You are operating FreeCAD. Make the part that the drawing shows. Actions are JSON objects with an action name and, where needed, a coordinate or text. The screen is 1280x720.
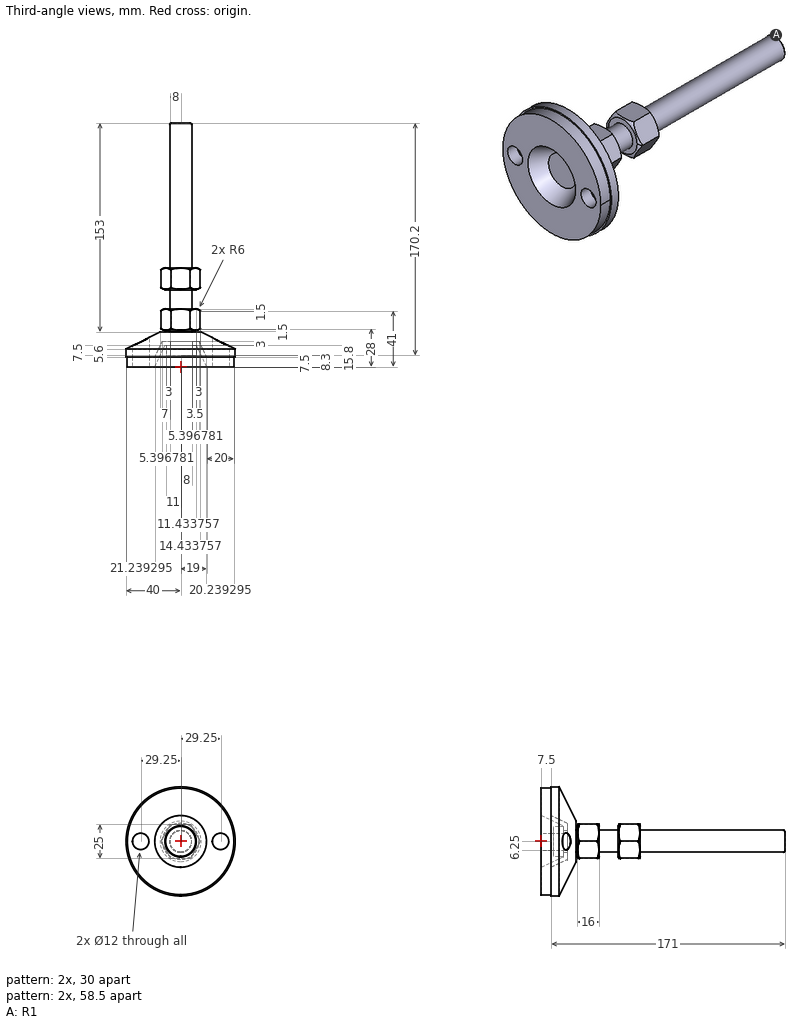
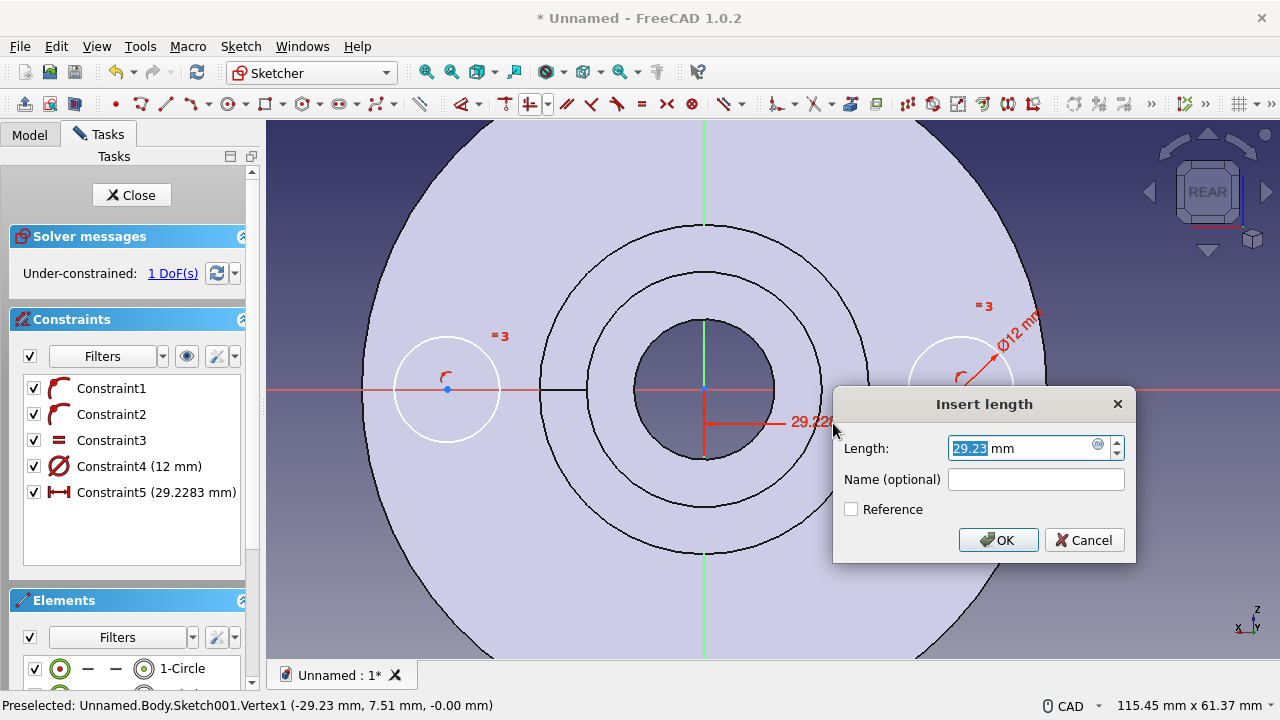
{"action": "type", "text": "29.25"}
{"action": "key", "text": "Return"}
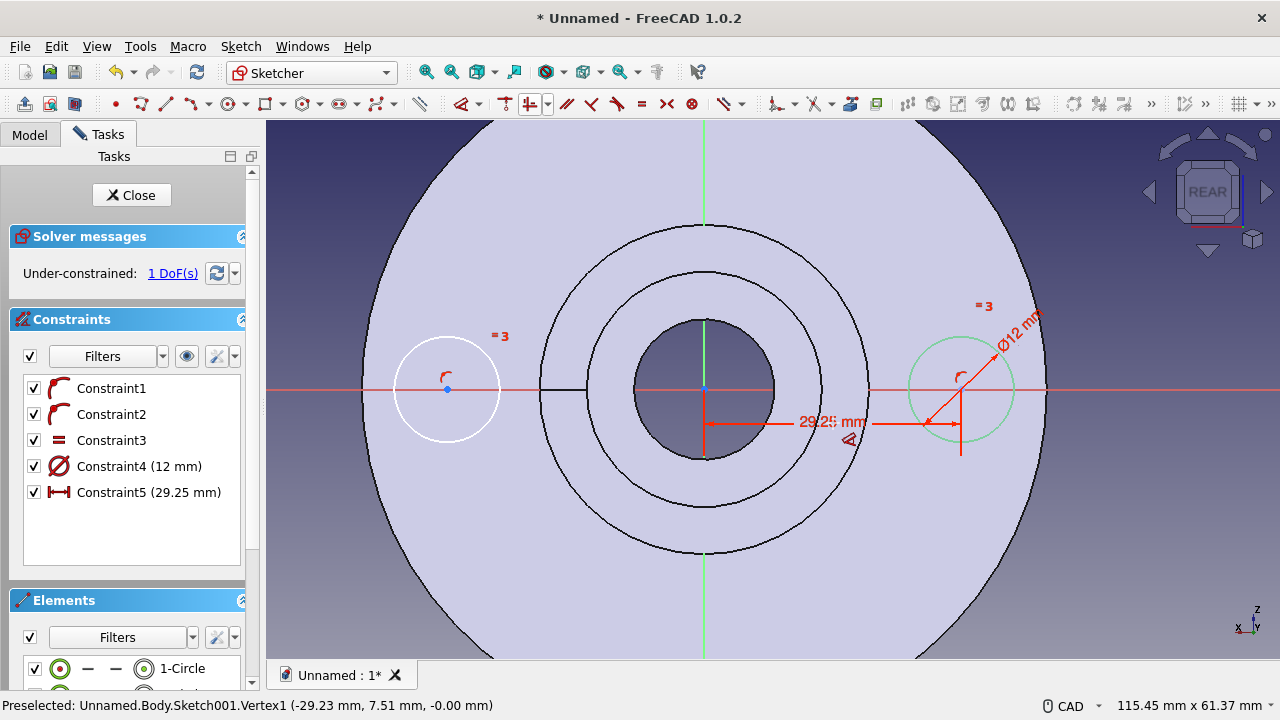
{"action": "left_click", "coordinate": [447, 389]}
{"action": "left_click", "coordinate": [576, 423]}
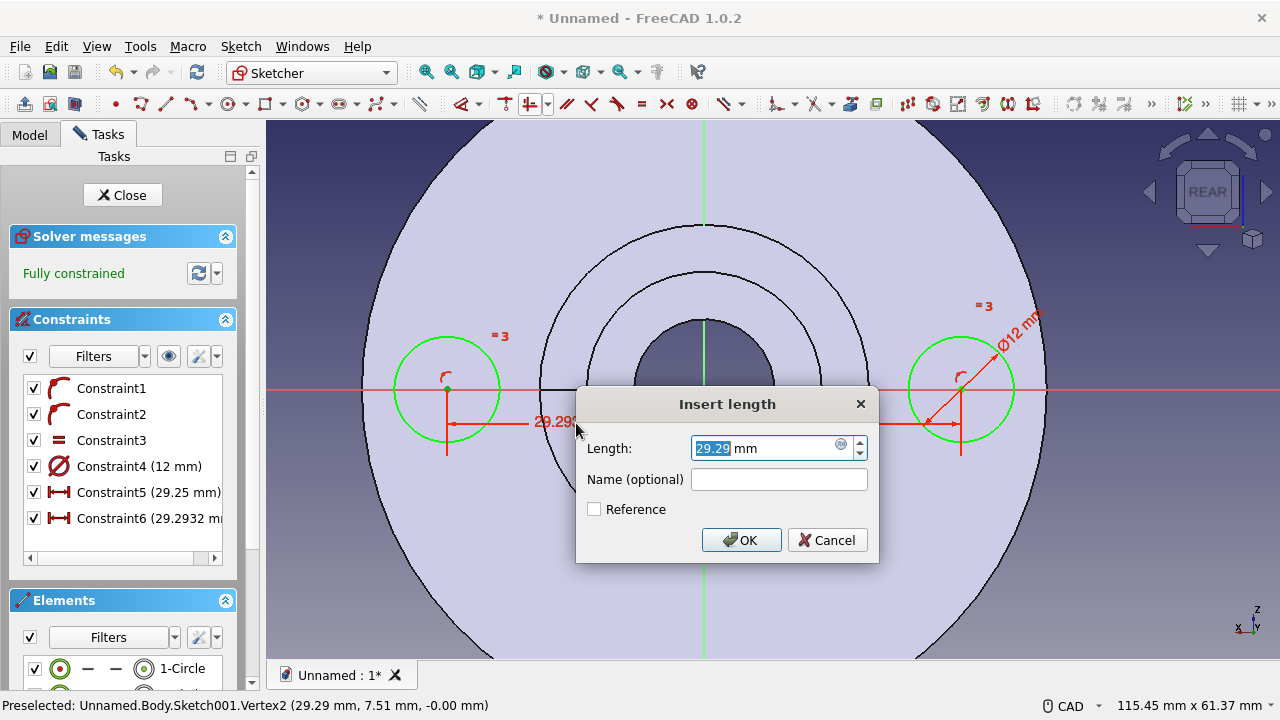
{"action": "type", "text": "29.25"}
{"action": "key", "text": "Return"}
{"action": "key", "text": "Escape"}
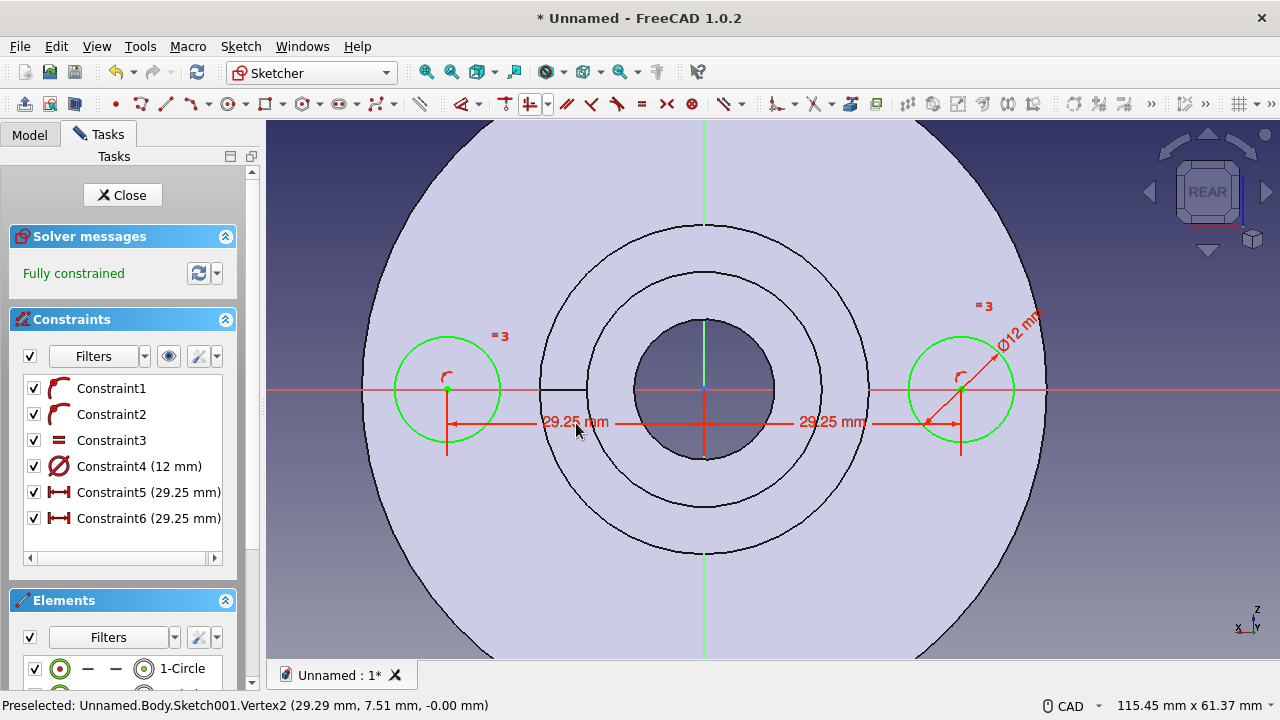
{"action": "left_click", "coordinate": [123, 195]}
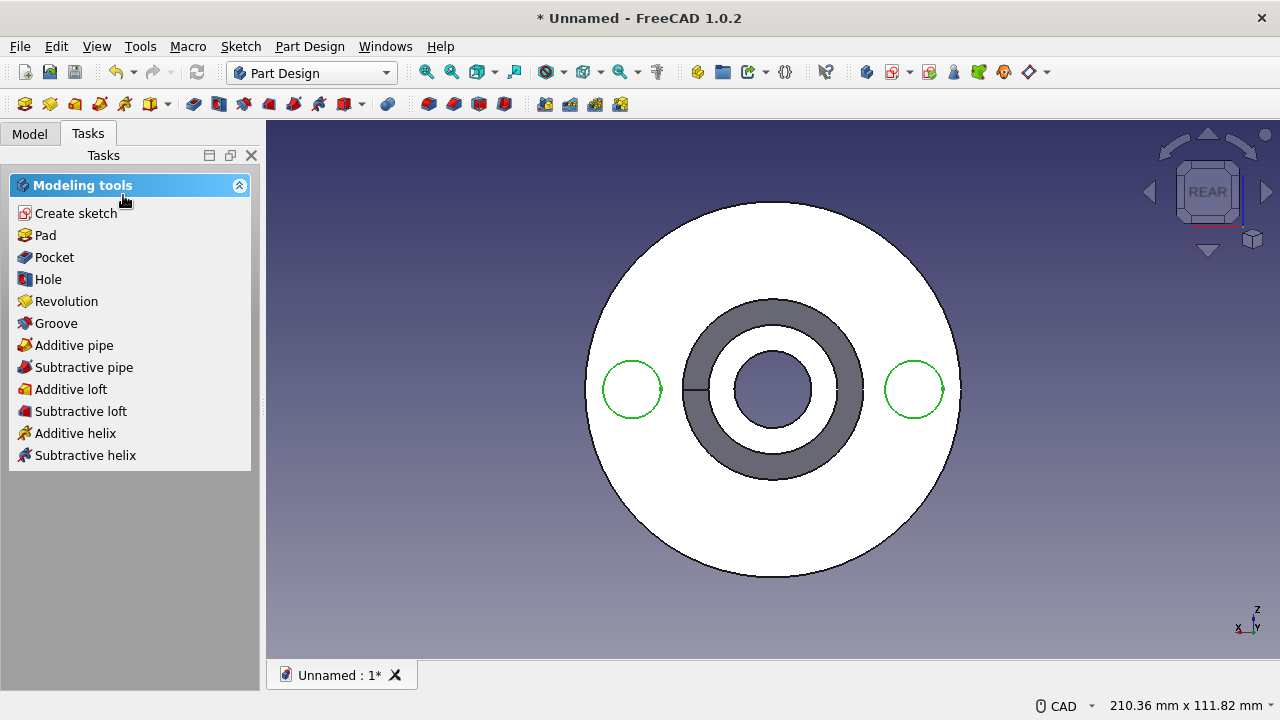
{"action": "left_click", "coordinate": [219, 104]}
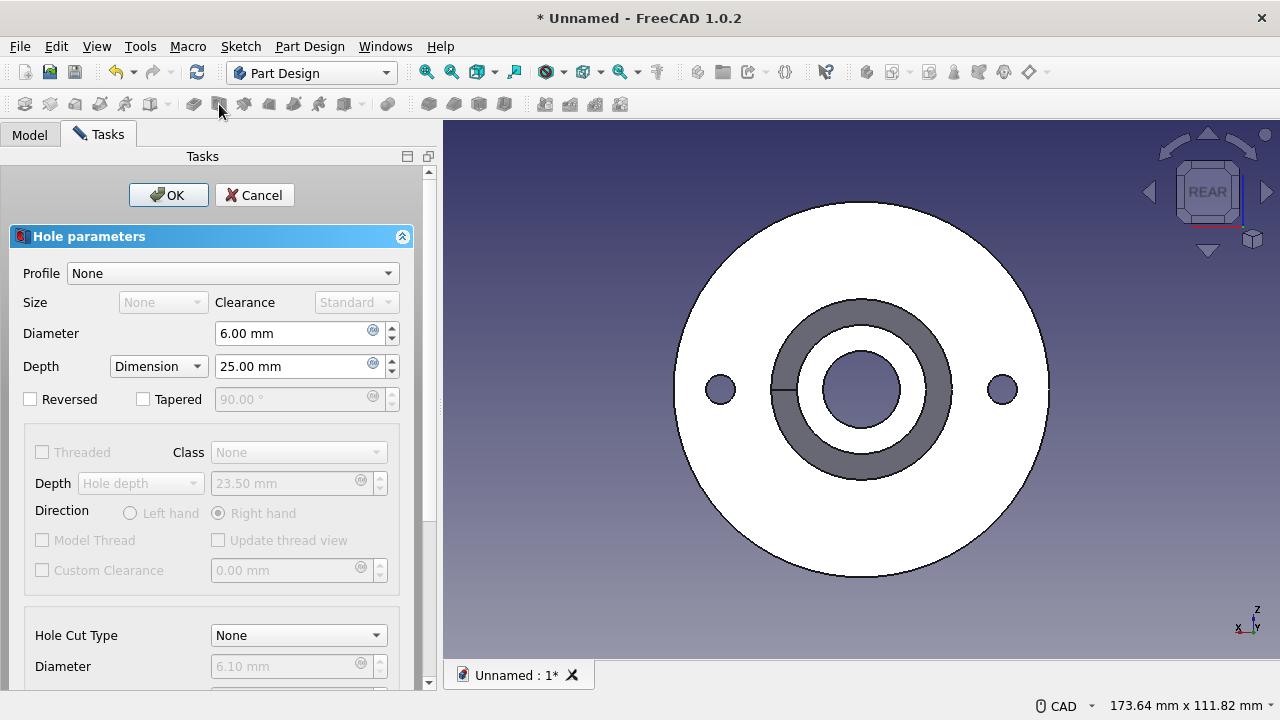
{"action": "triple_click", "coordinate": [300, 334]}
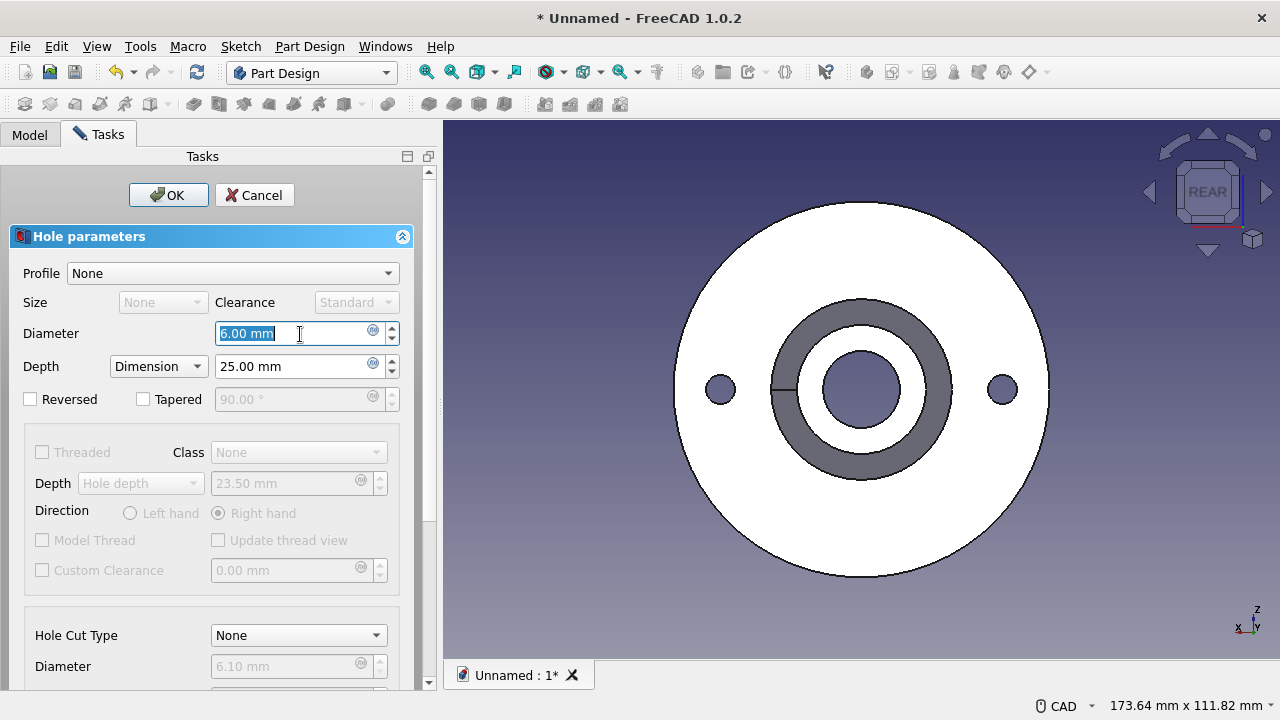
{"action": "type", "text": "12"}
{"action": "key", "text": "Tab"}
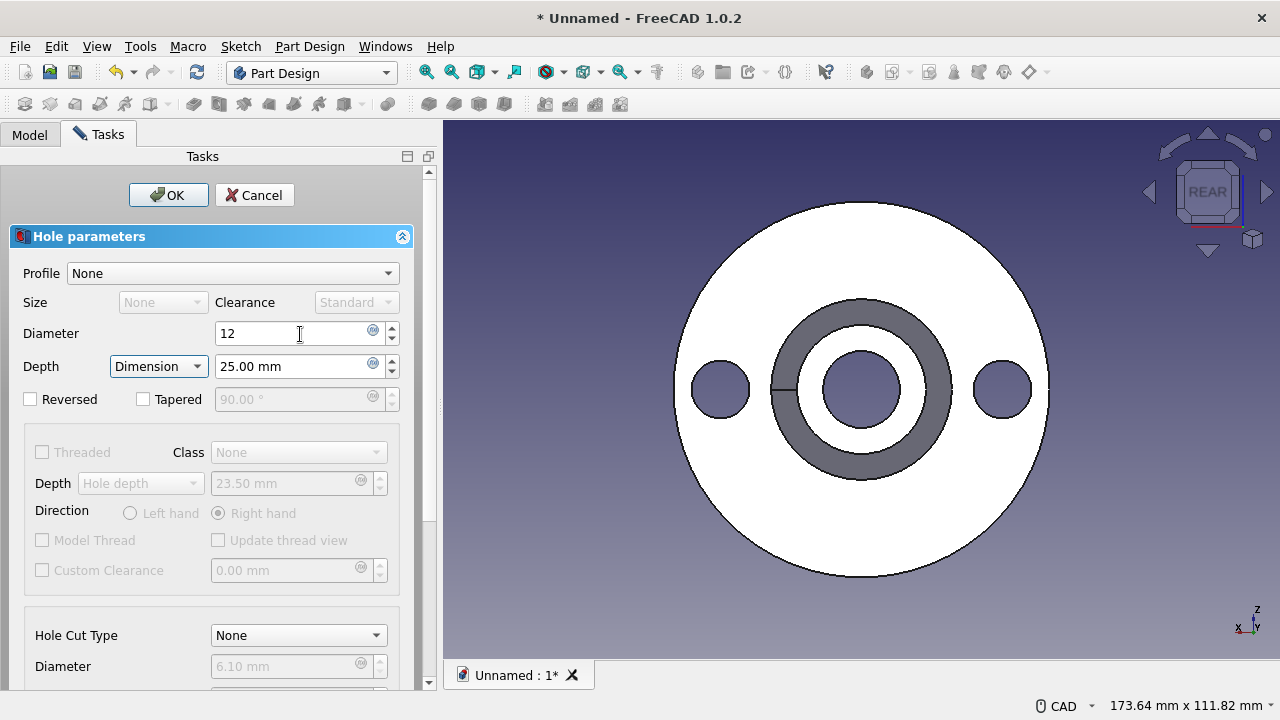
{"action": "left_click", "coordinate": [160, 366]}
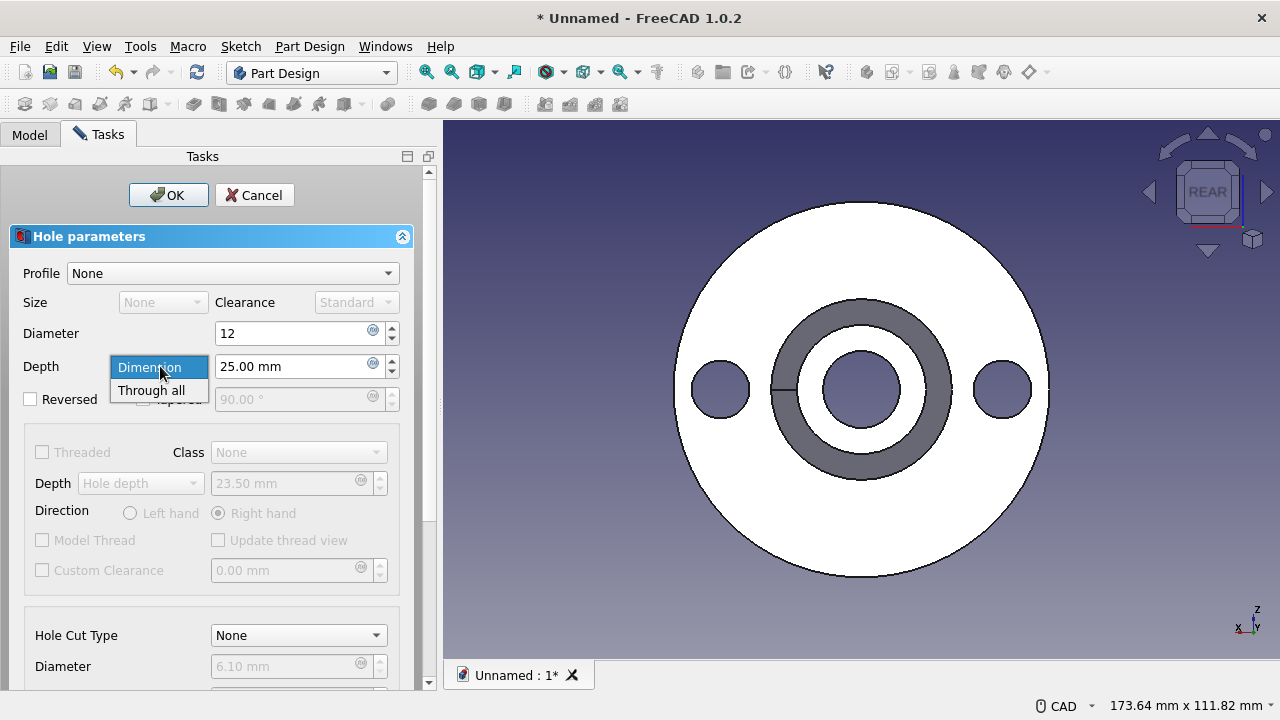
{"action": "left_click", "coordinate": [158, 390]}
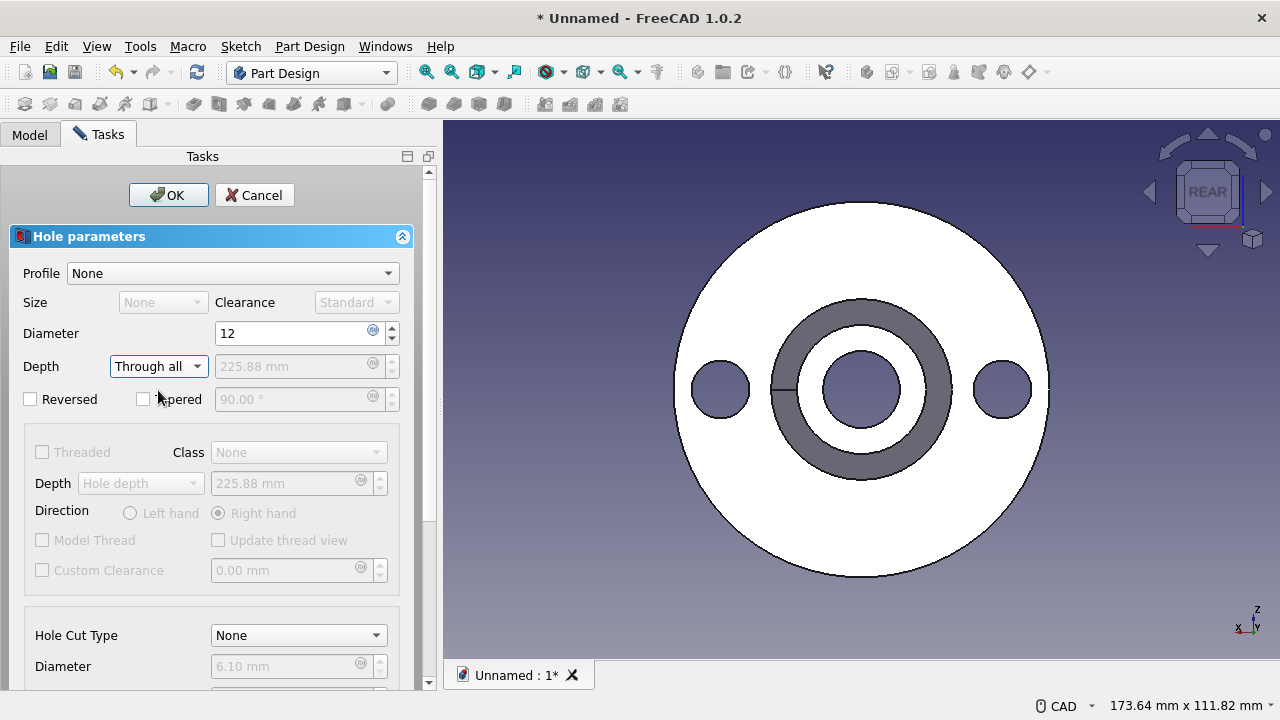
{"action": "left_click", "coordinate": [169, 195]}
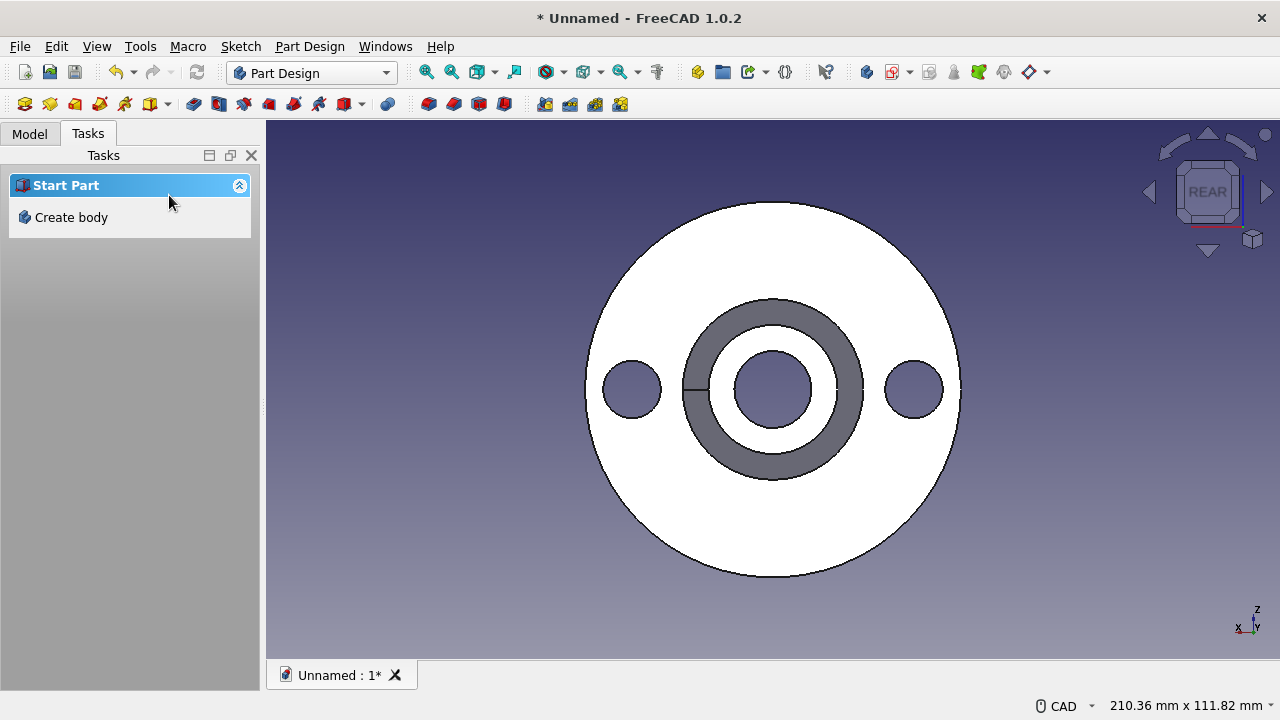
{"action": "left_click", "coordinate": [867, 72]}